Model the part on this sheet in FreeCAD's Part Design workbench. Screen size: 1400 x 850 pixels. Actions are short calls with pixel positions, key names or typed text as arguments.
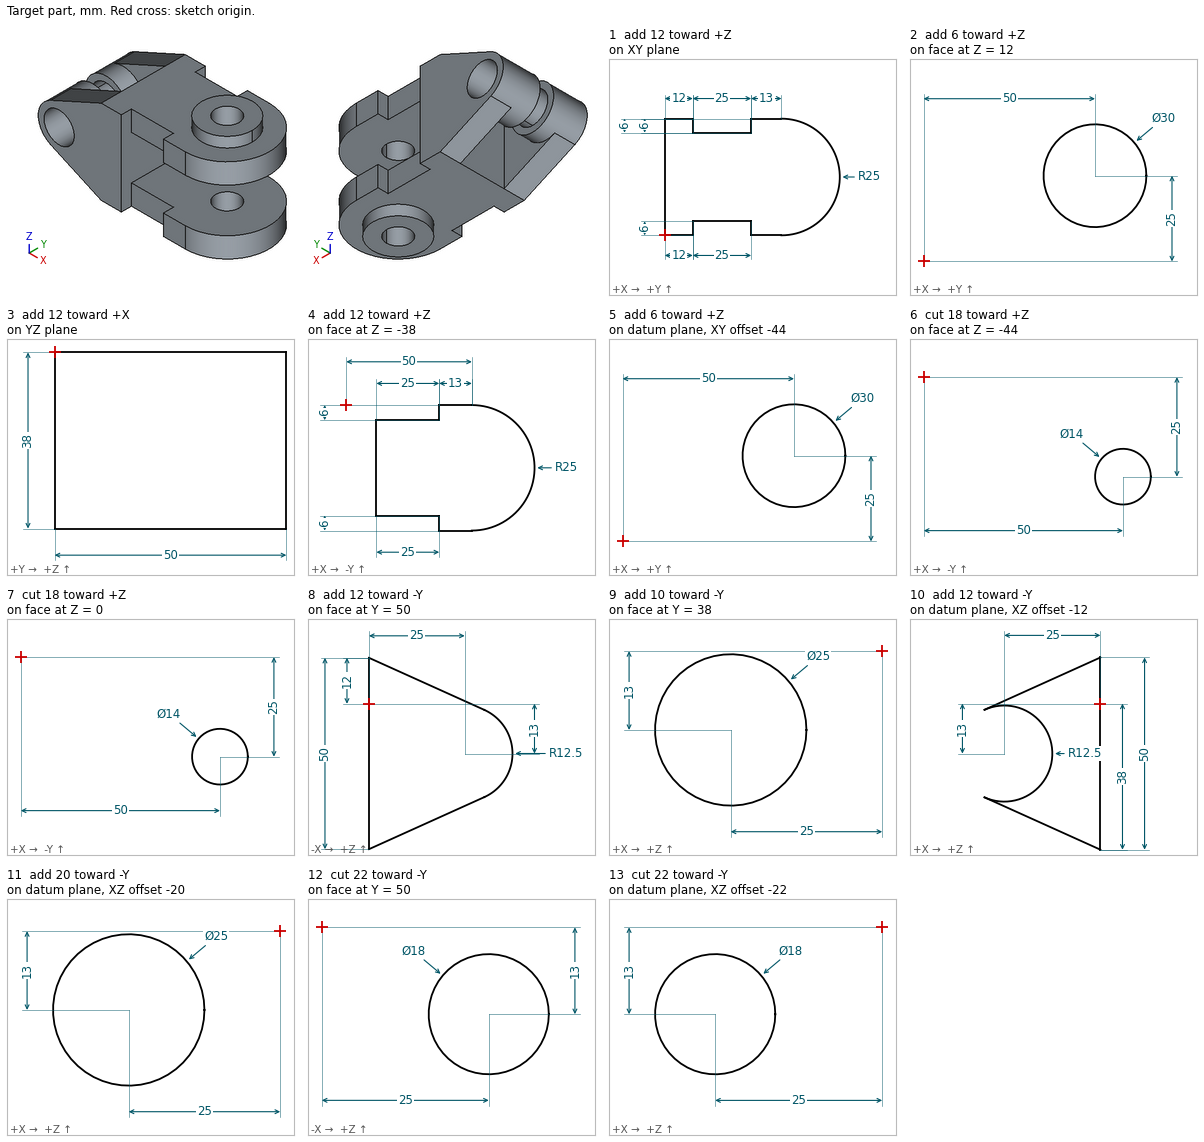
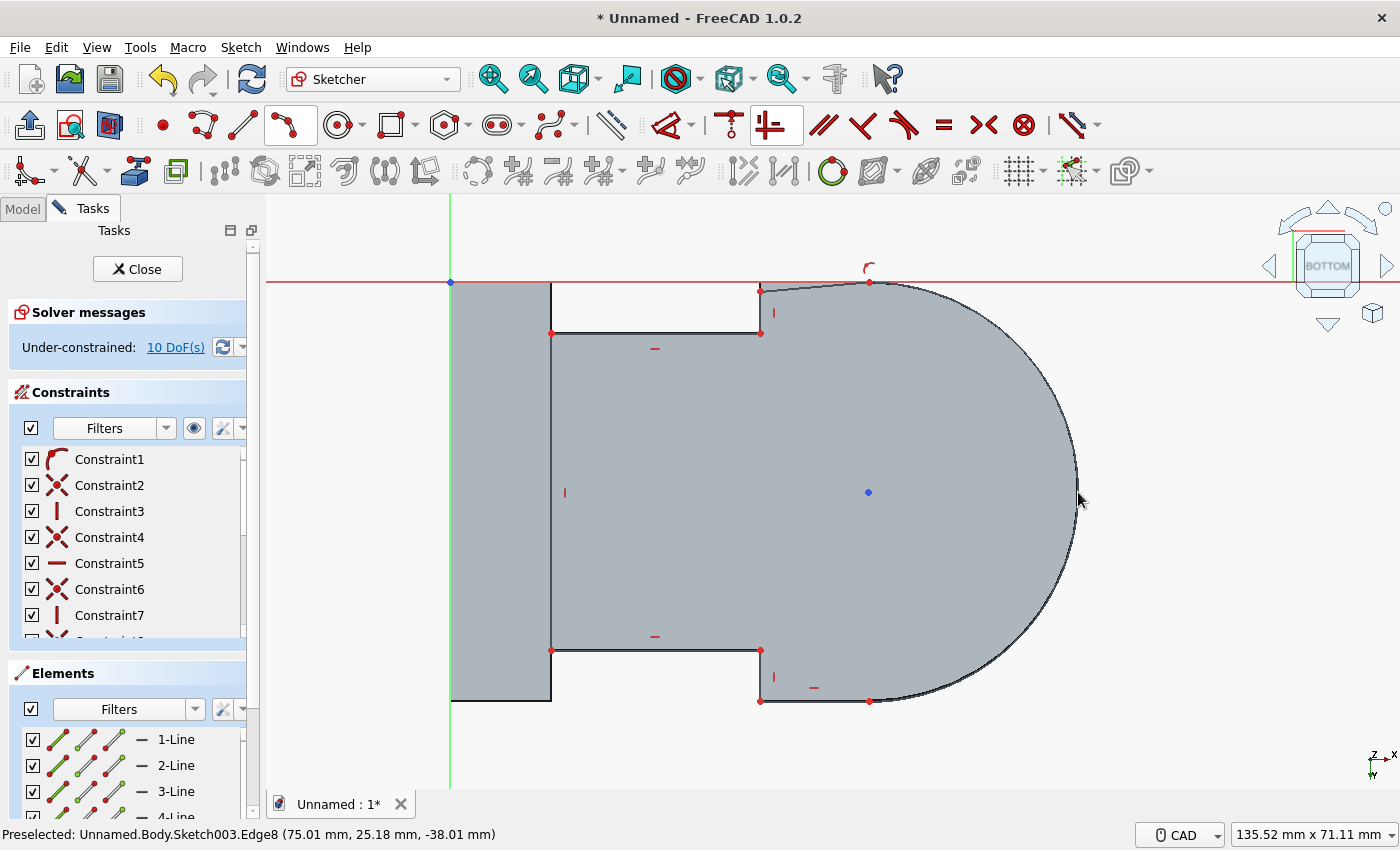
click(836, 285)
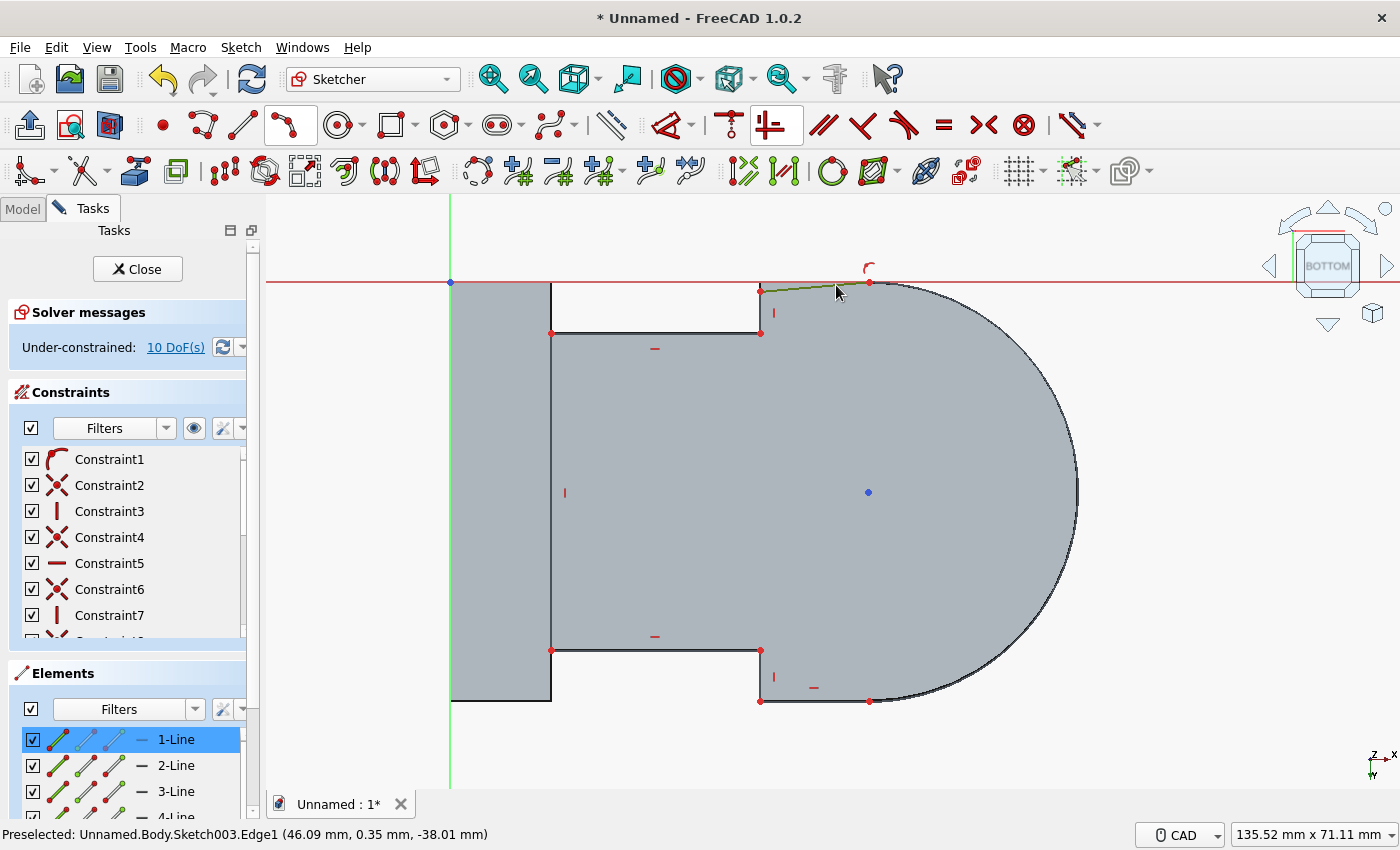
click(1038, 615)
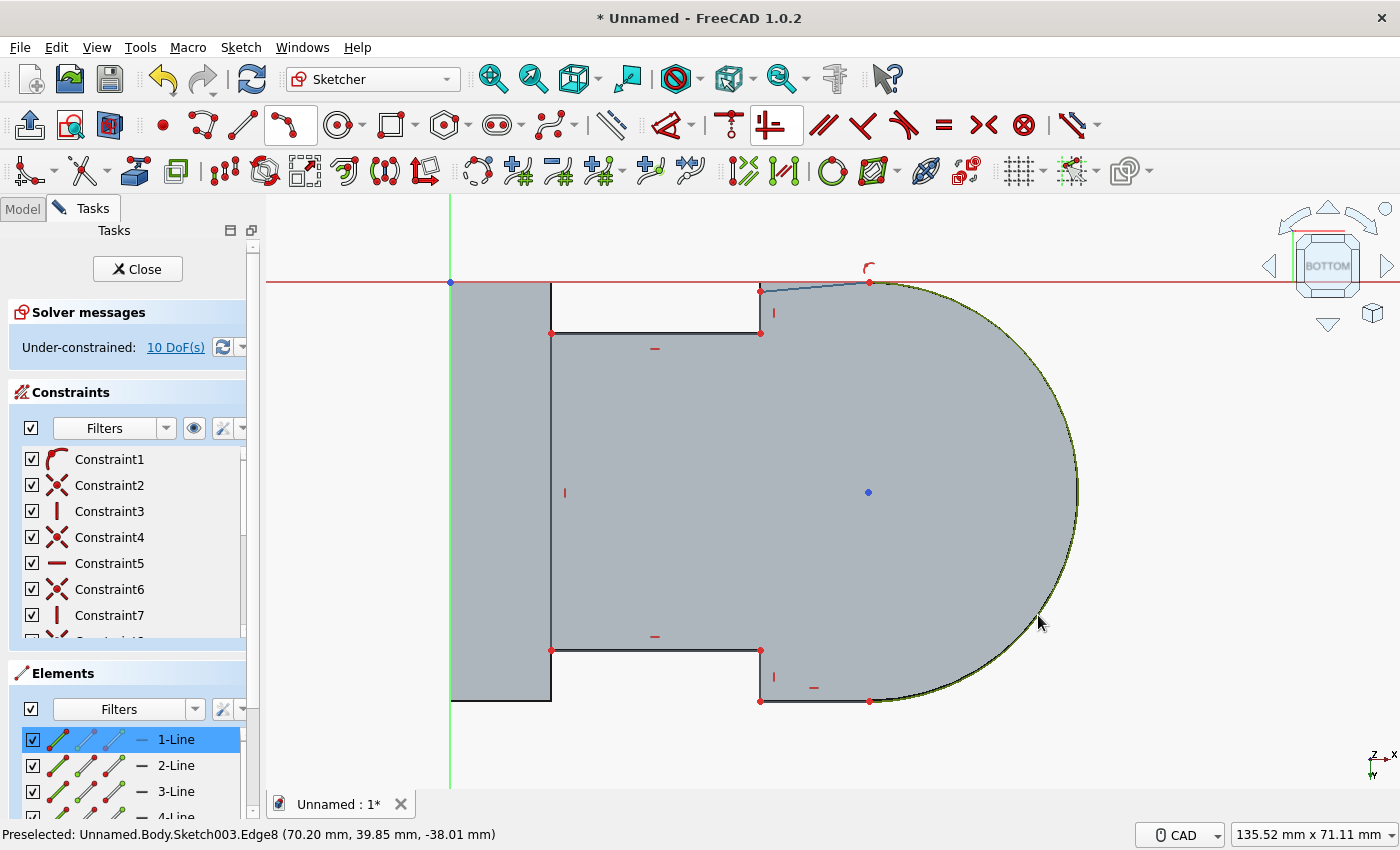
click(904, 126)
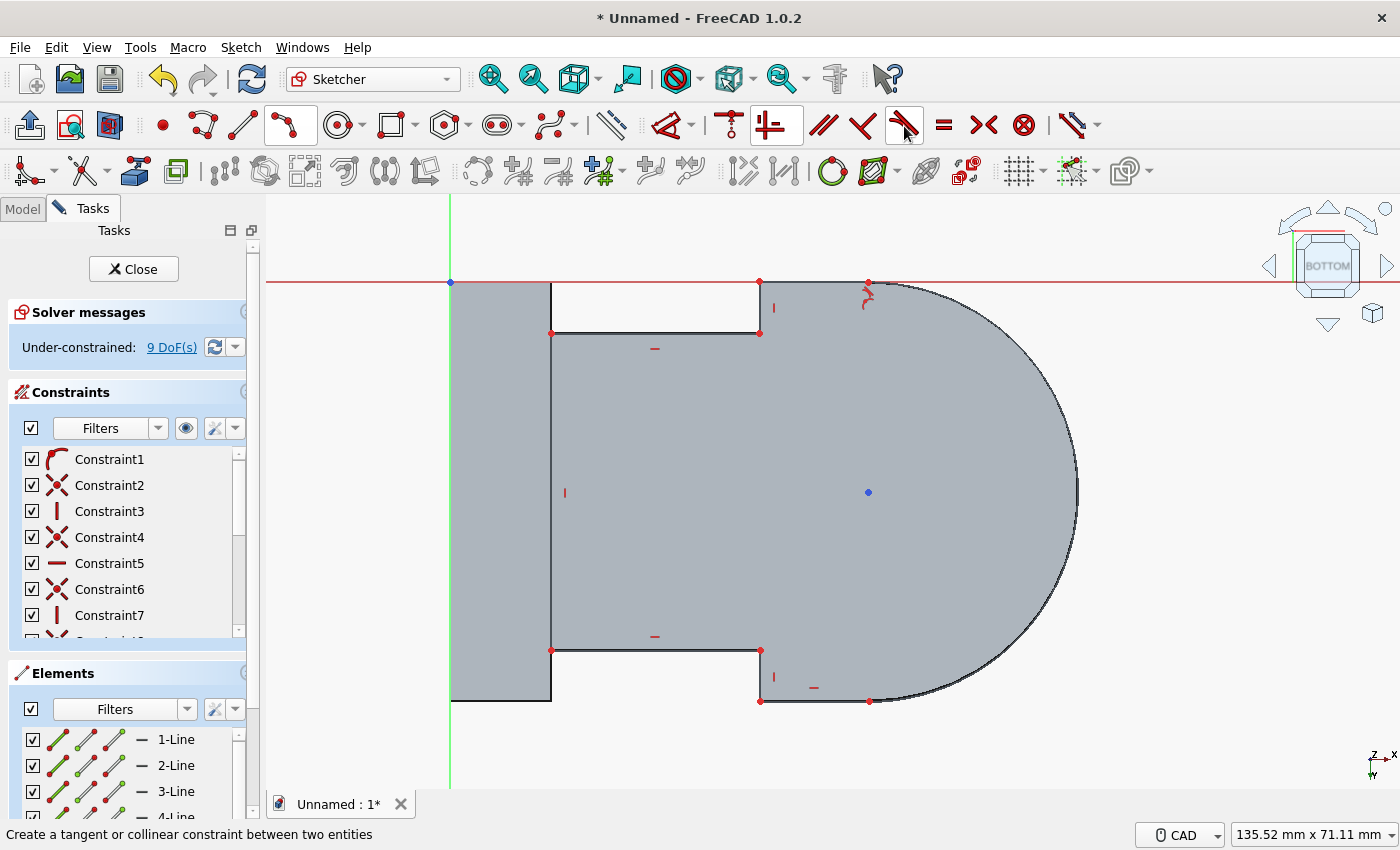
click(793, 702)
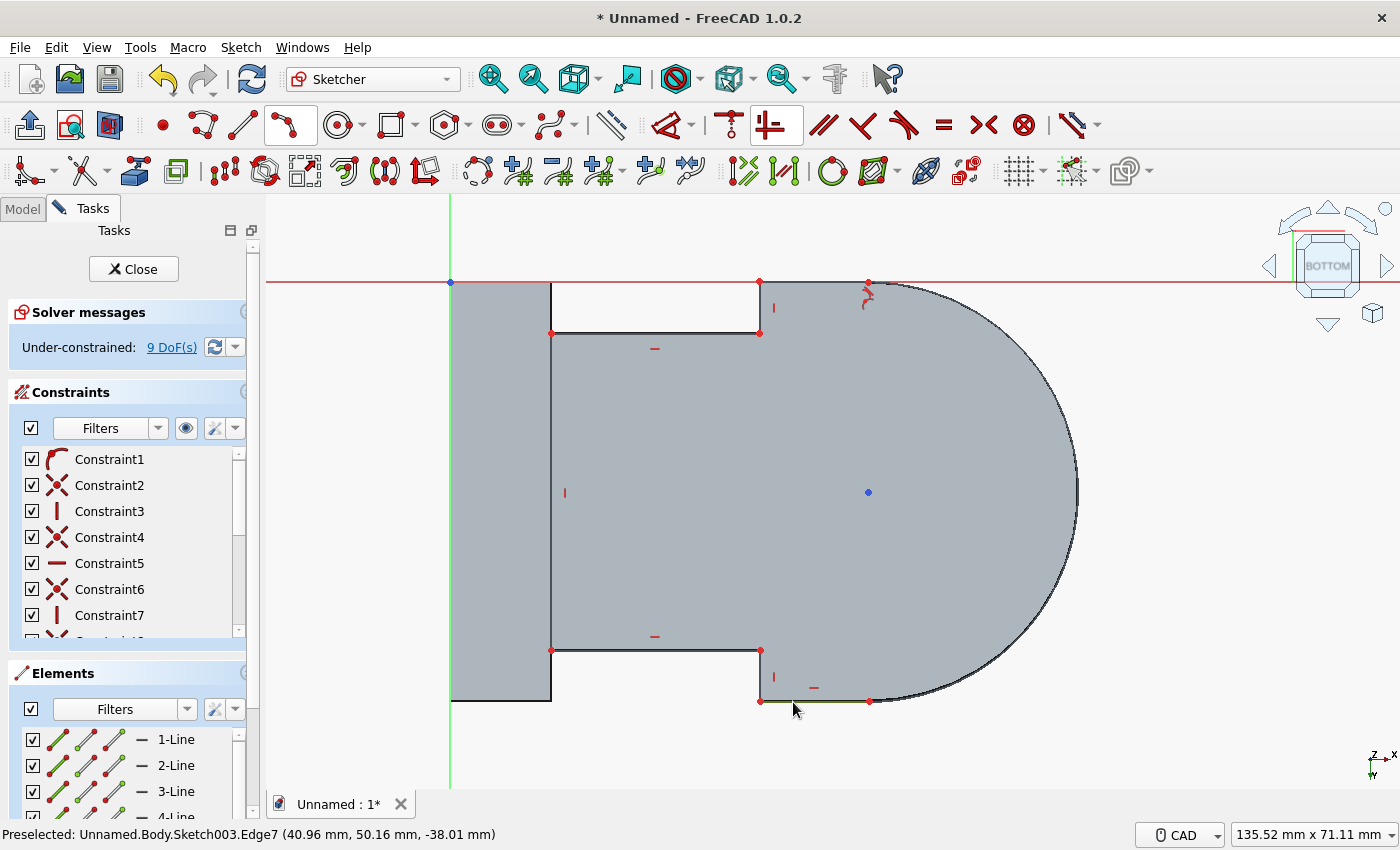
click(1038, 615)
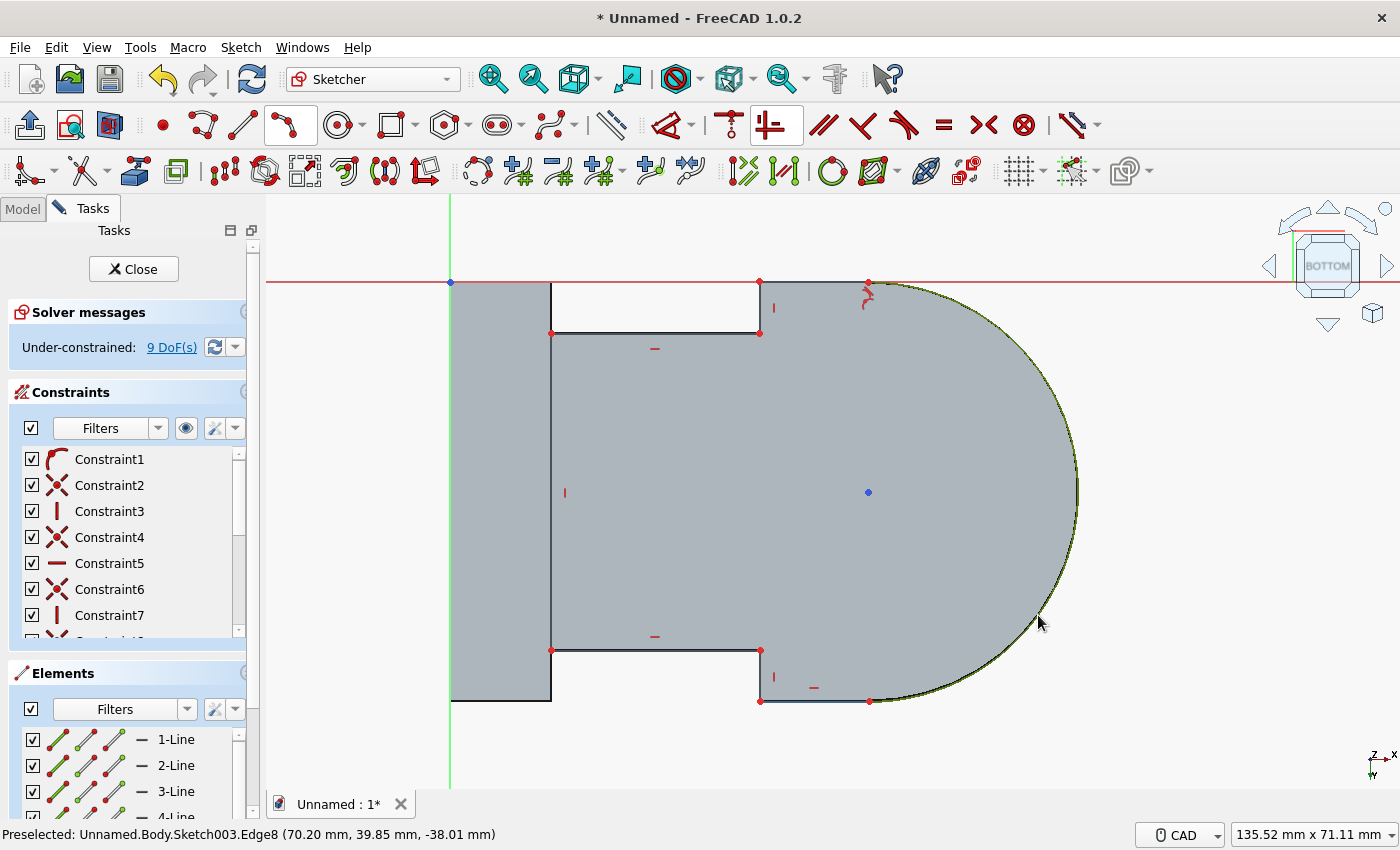
click(904, 126)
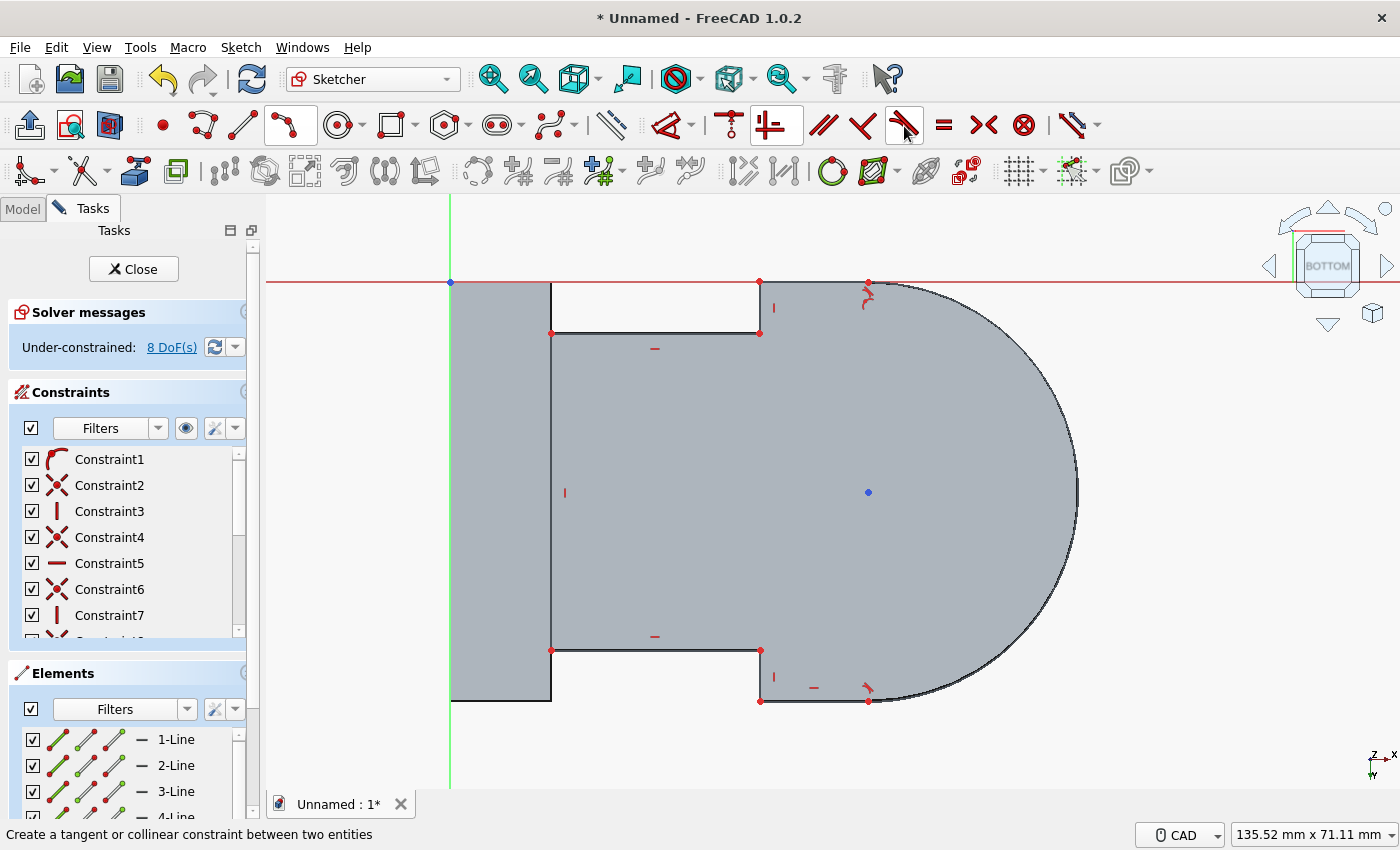
click(836, 282)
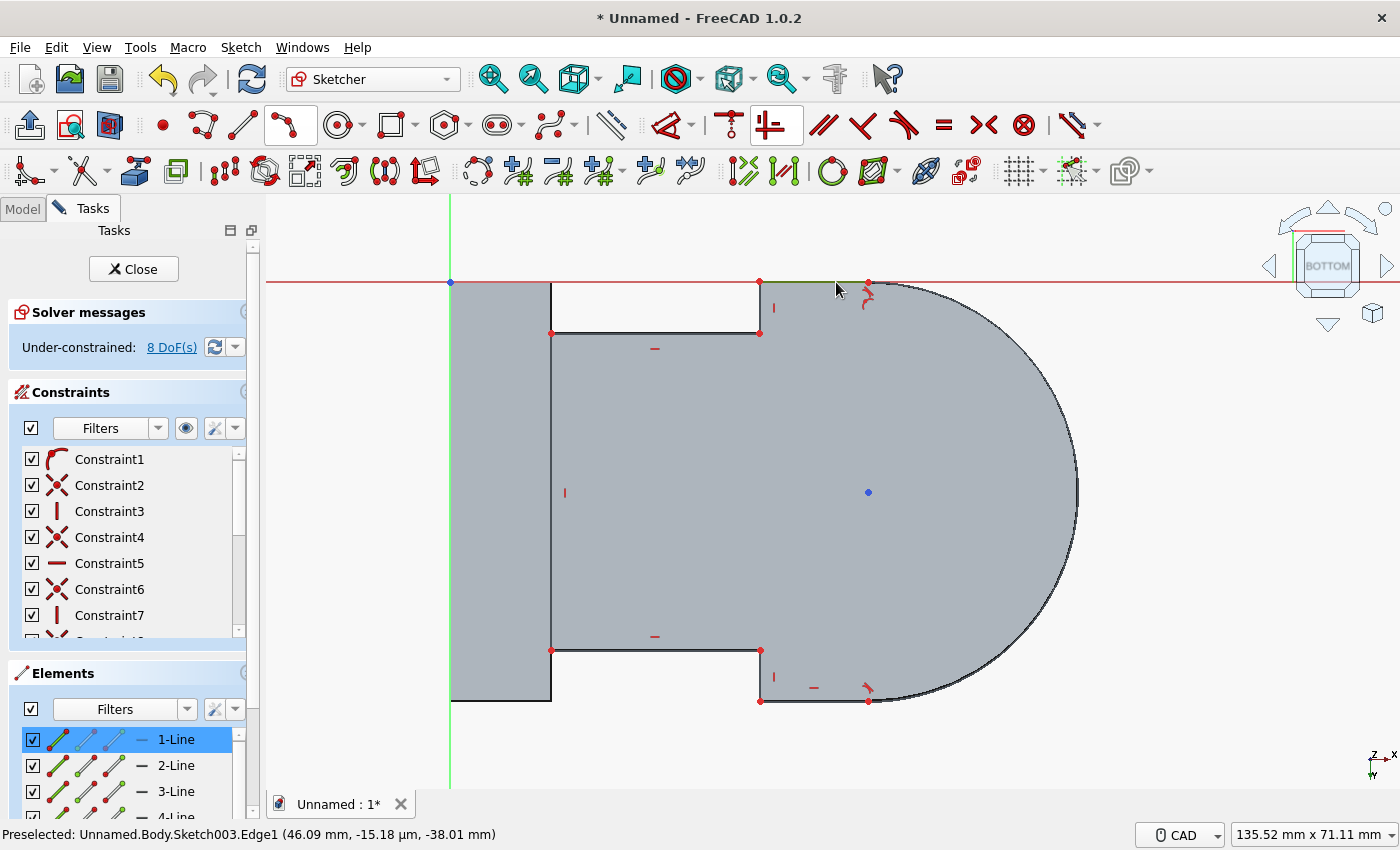
click(798, 126)